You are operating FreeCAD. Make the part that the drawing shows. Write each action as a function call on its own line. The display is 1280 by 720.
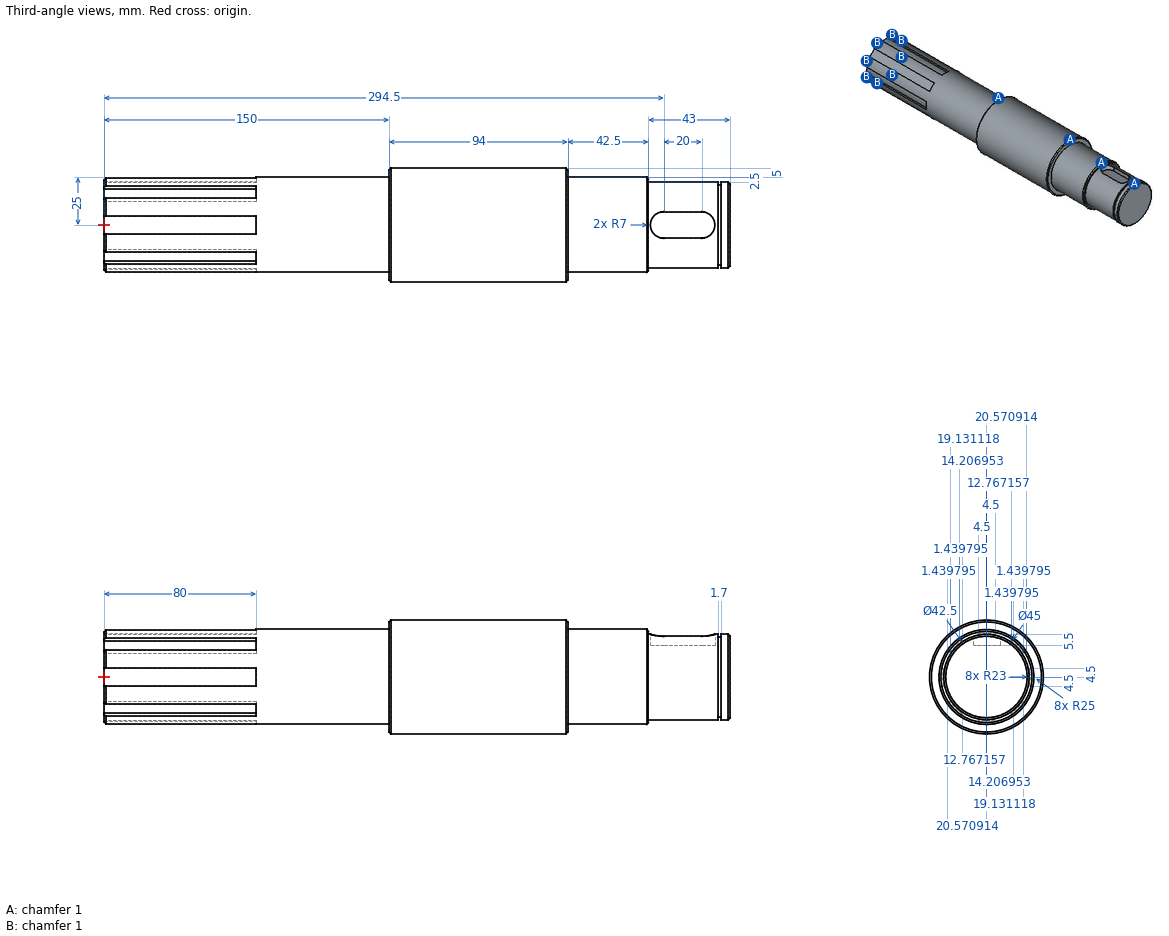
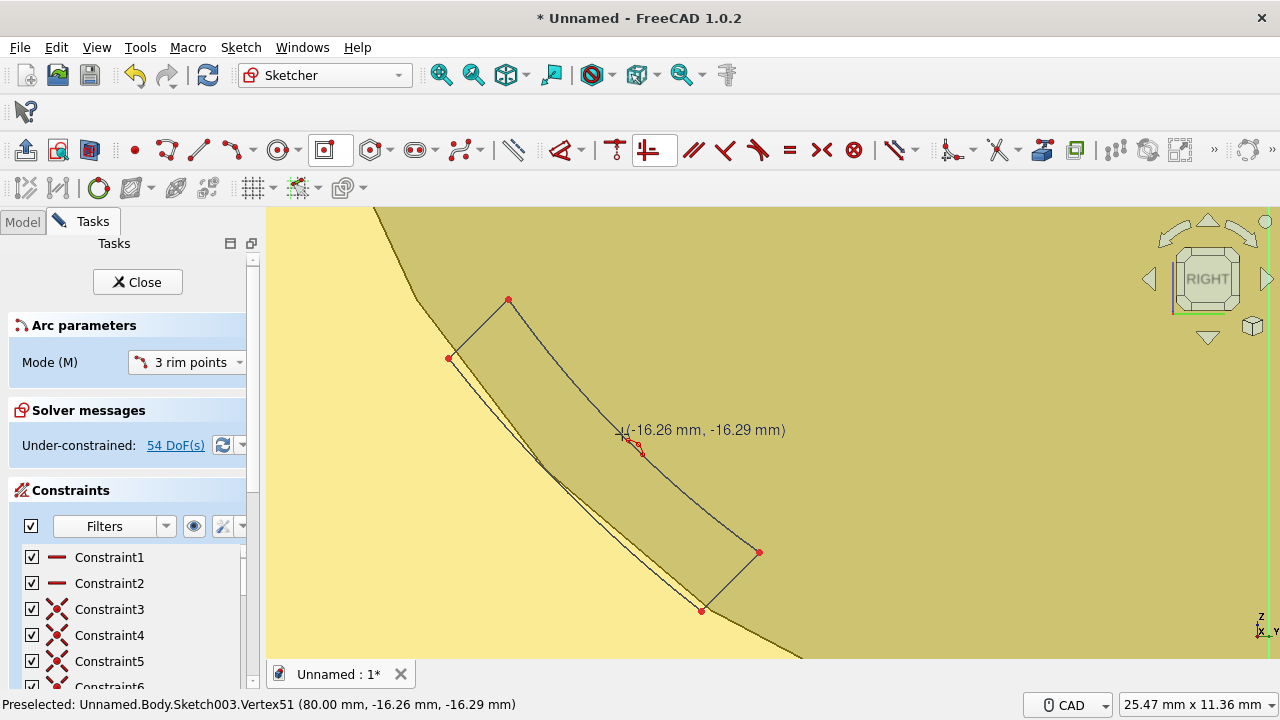
click(200, 150)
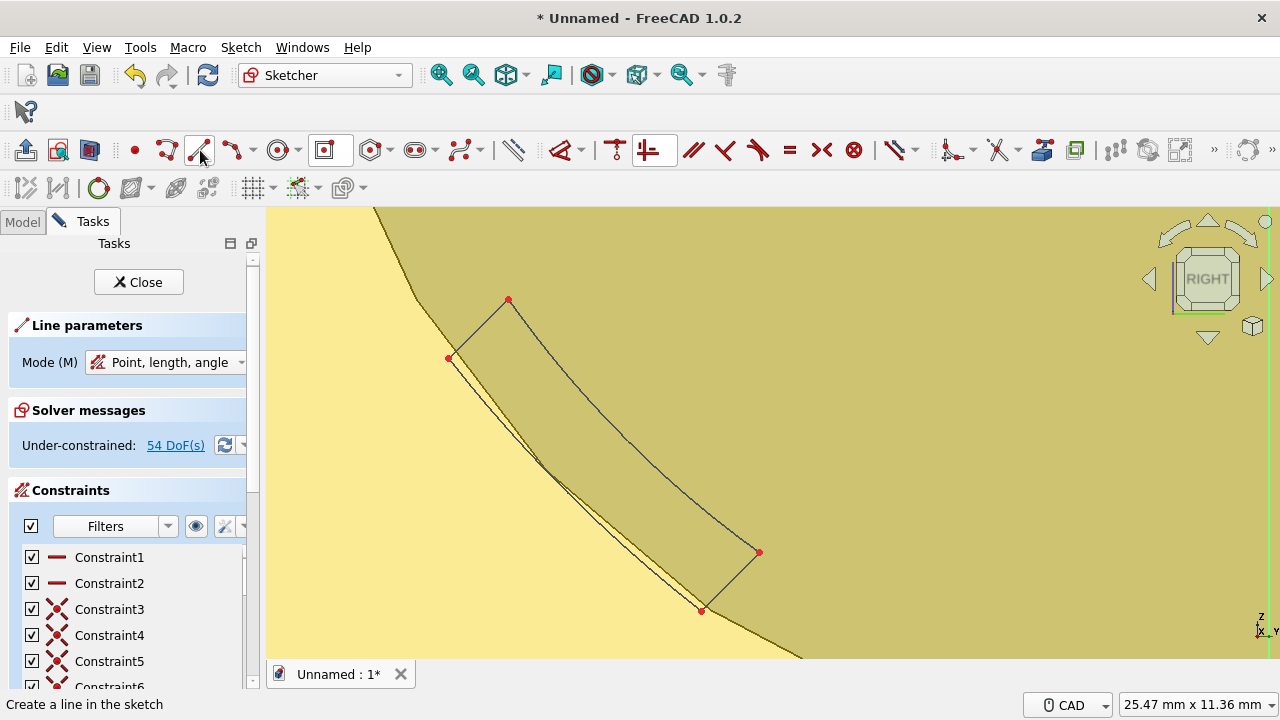
scroll(616, 534, down, 10)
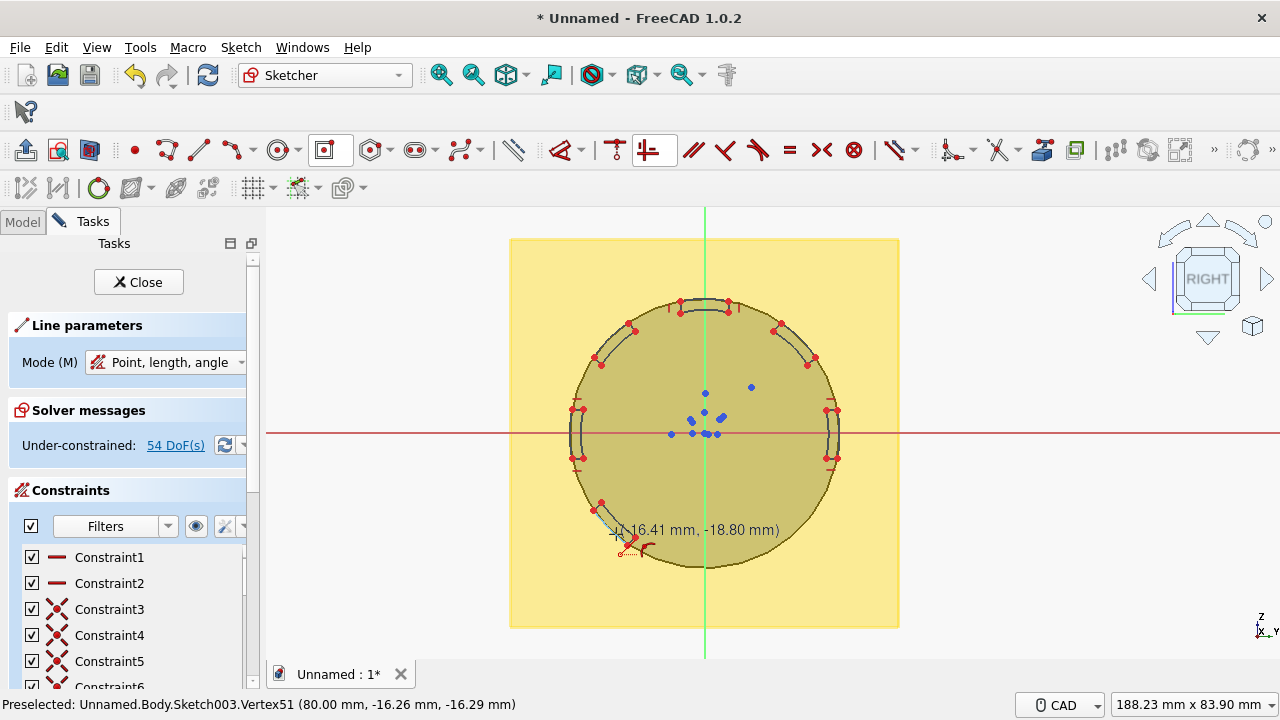
click(729, 555)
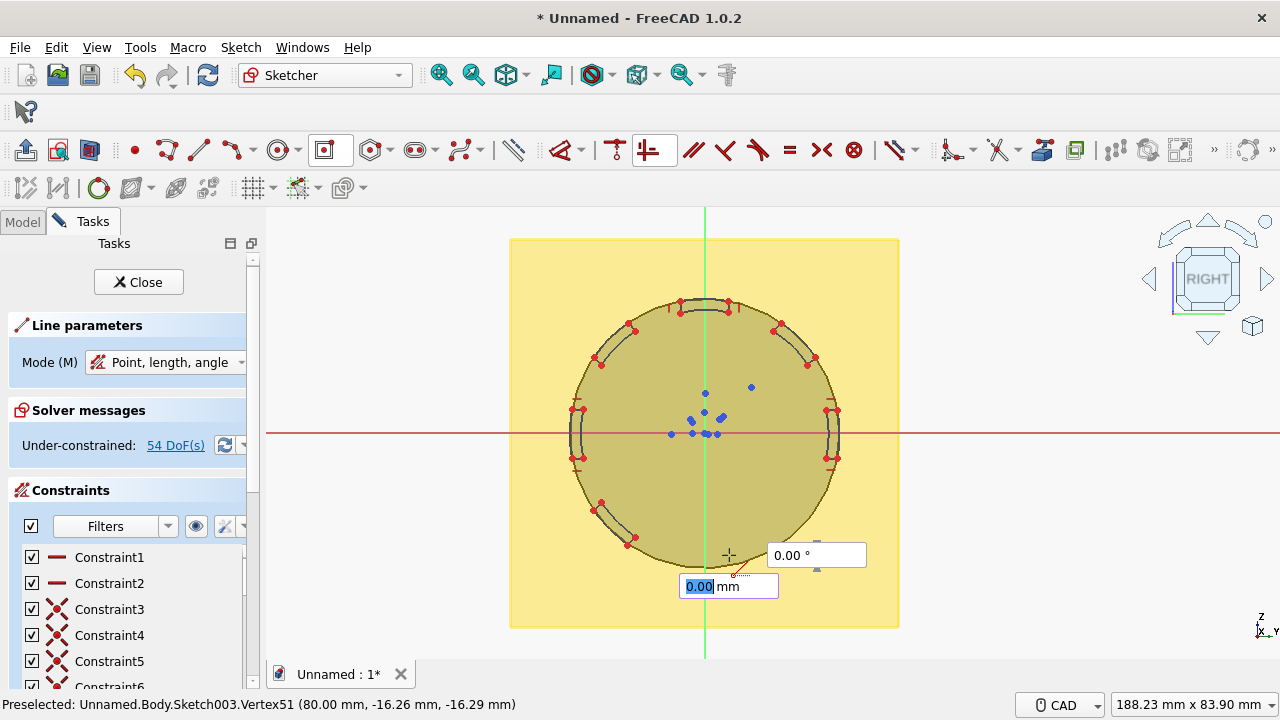
scroll(729, 566, up, 2)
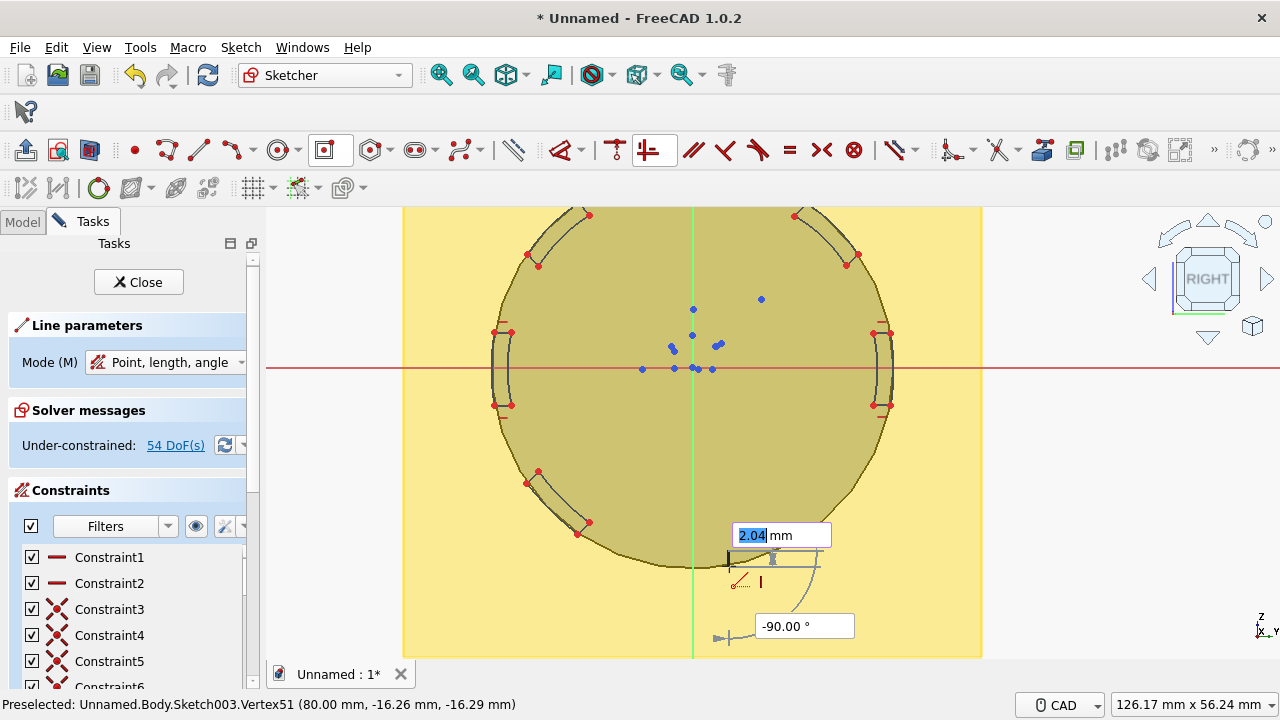
click(729, 566)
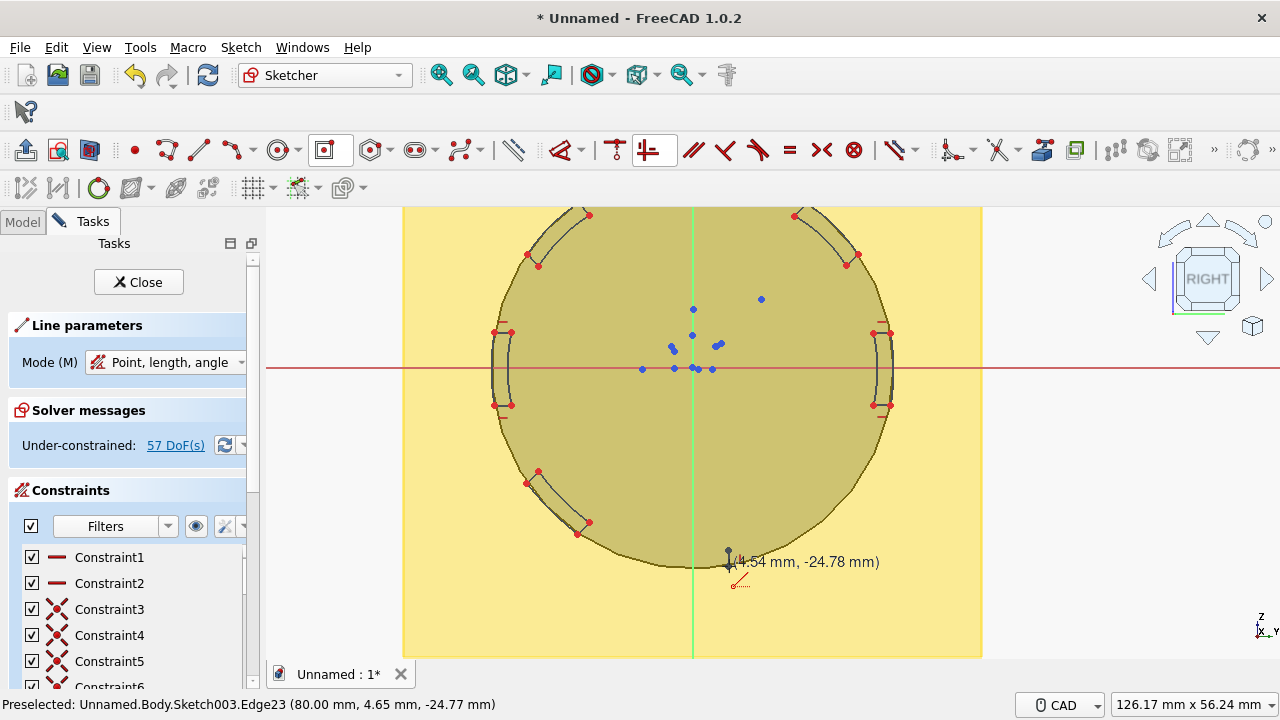
click(656, 566)
click(656, 549)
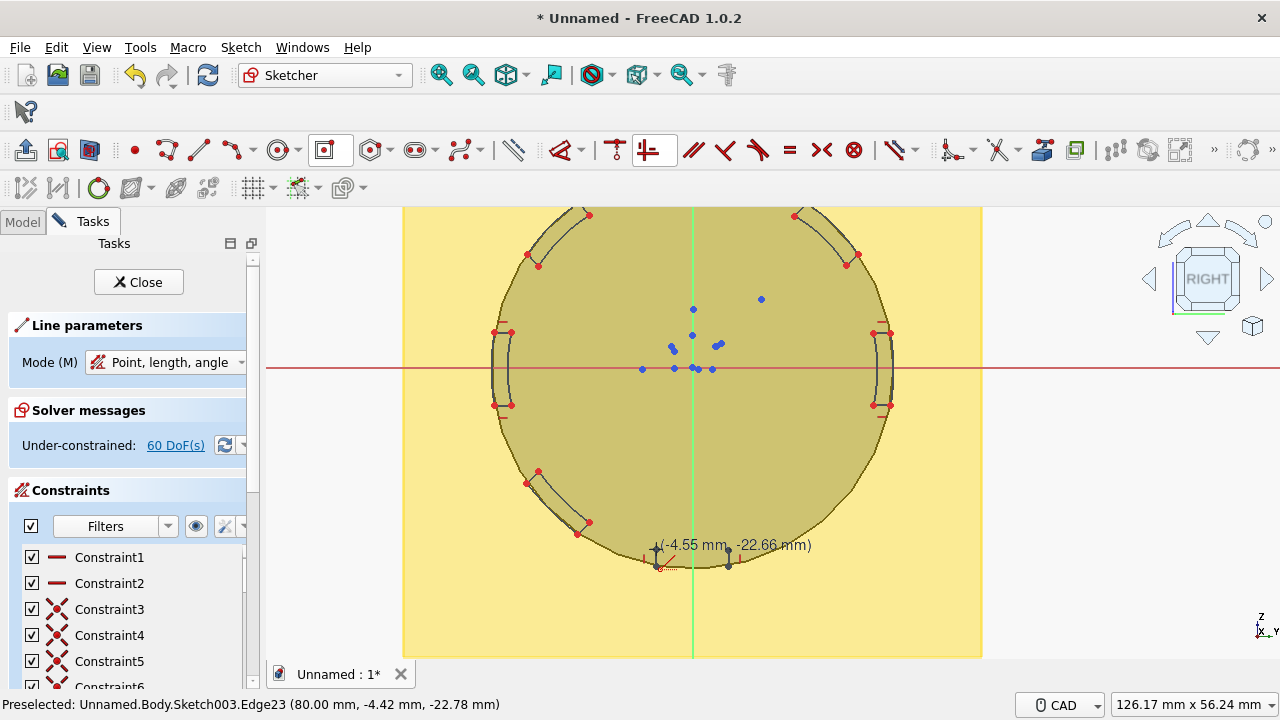
click(232, 150)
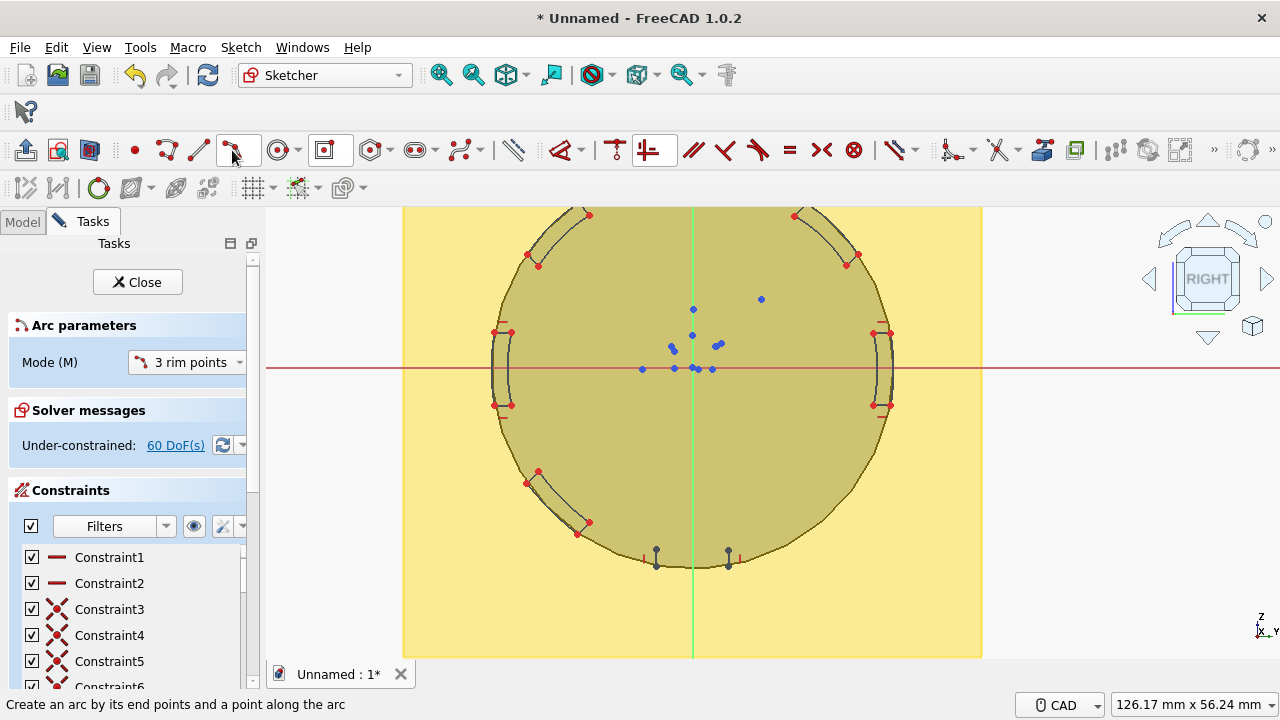
scroll(729, 566, up, 4)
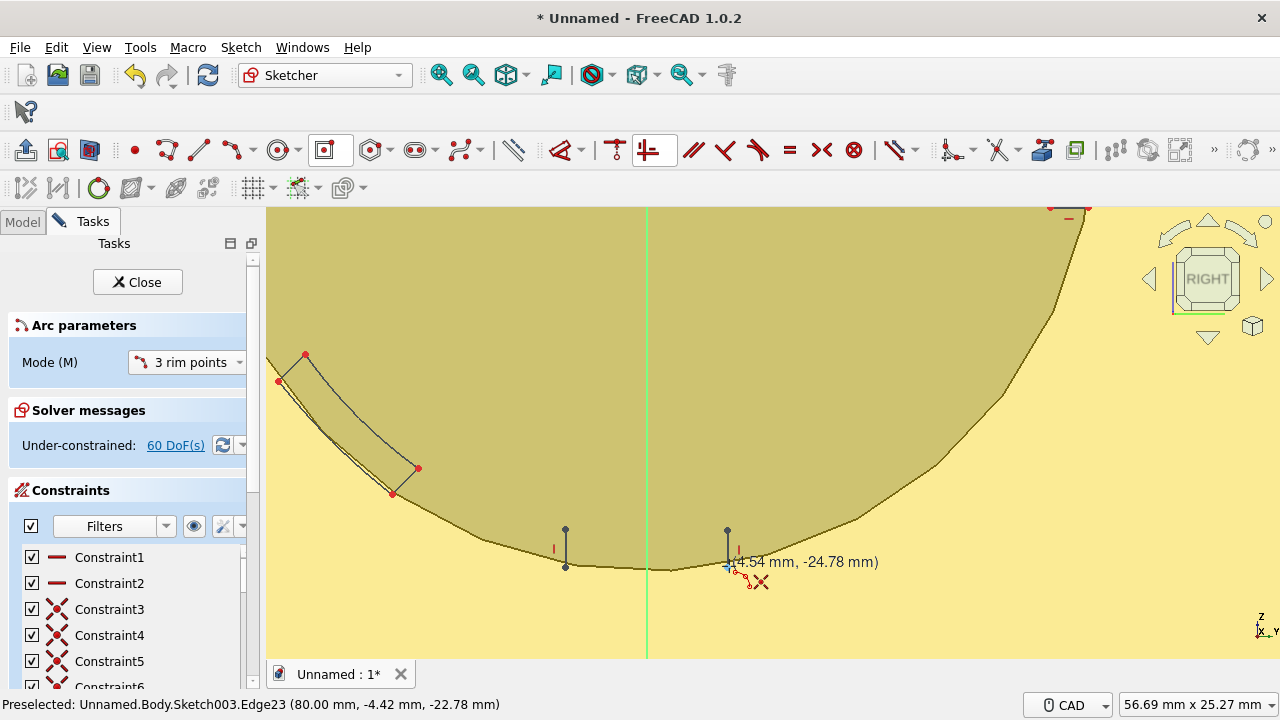
click(728, 567)
click(566, 567)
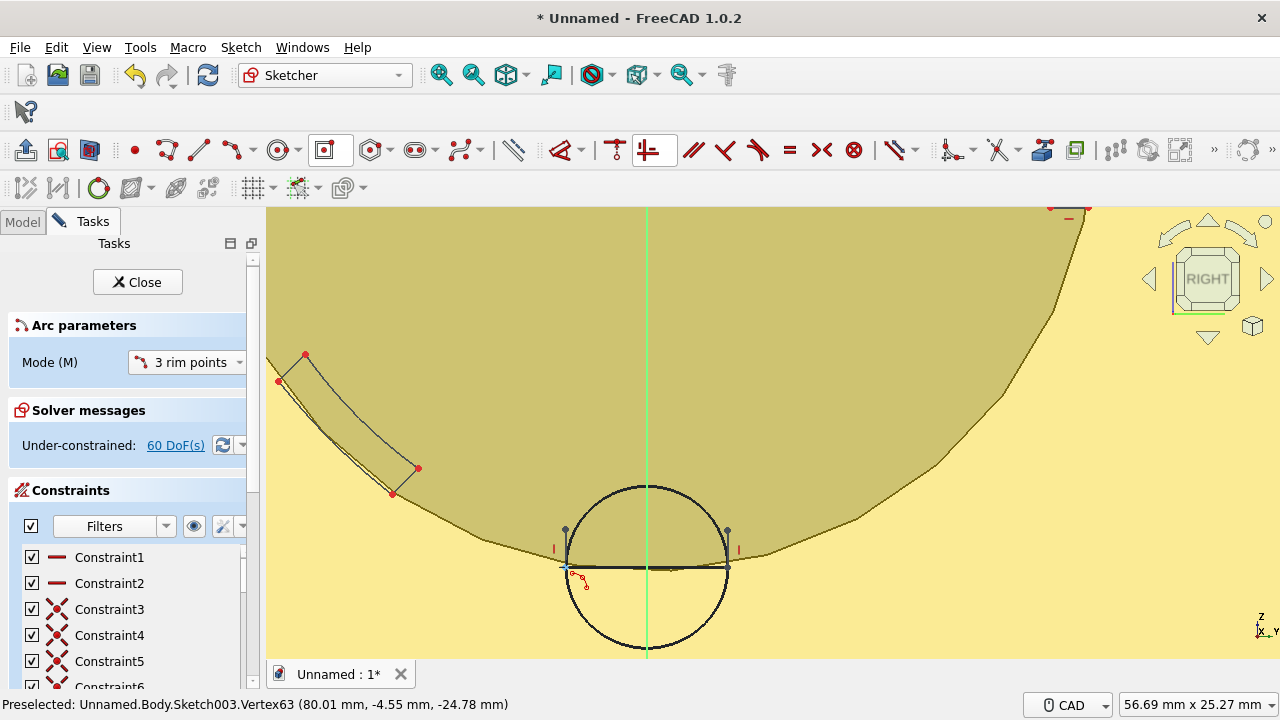
scroll(631, 571, up, 5)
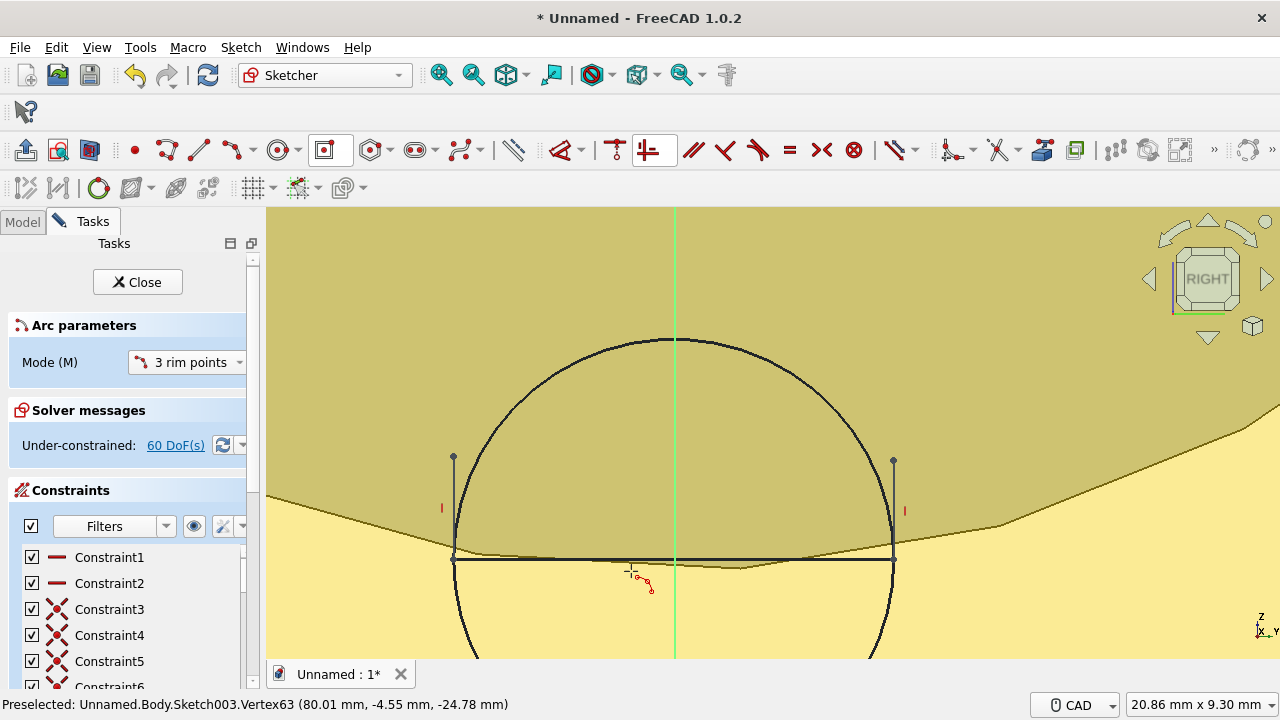
click(631, 570)